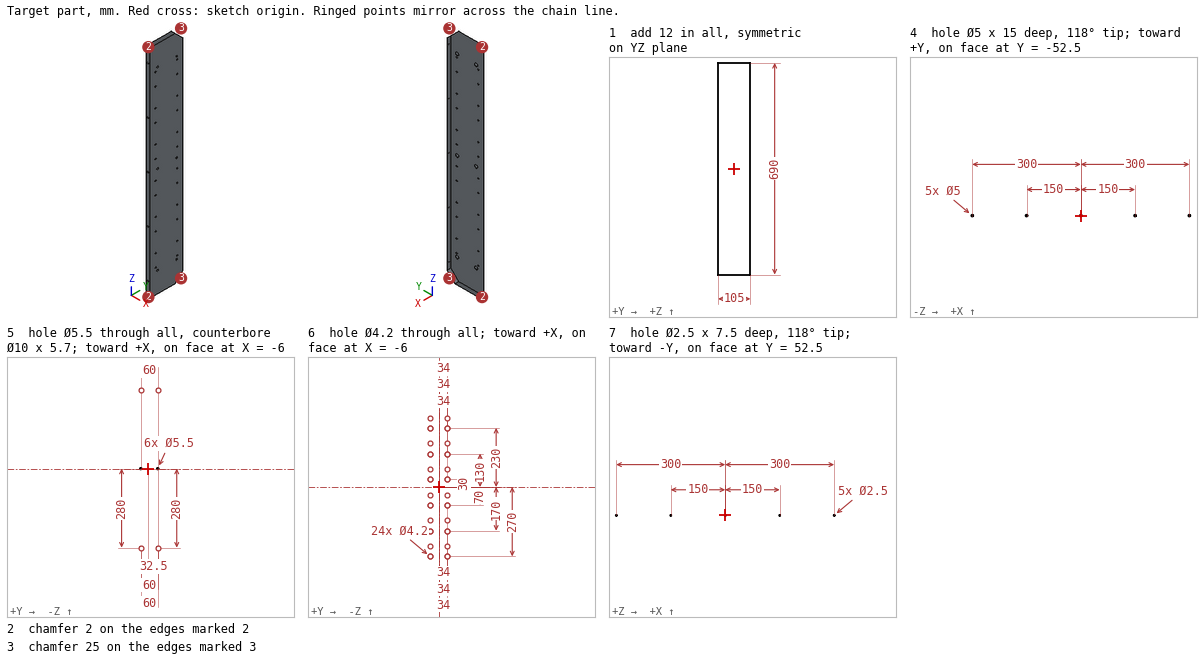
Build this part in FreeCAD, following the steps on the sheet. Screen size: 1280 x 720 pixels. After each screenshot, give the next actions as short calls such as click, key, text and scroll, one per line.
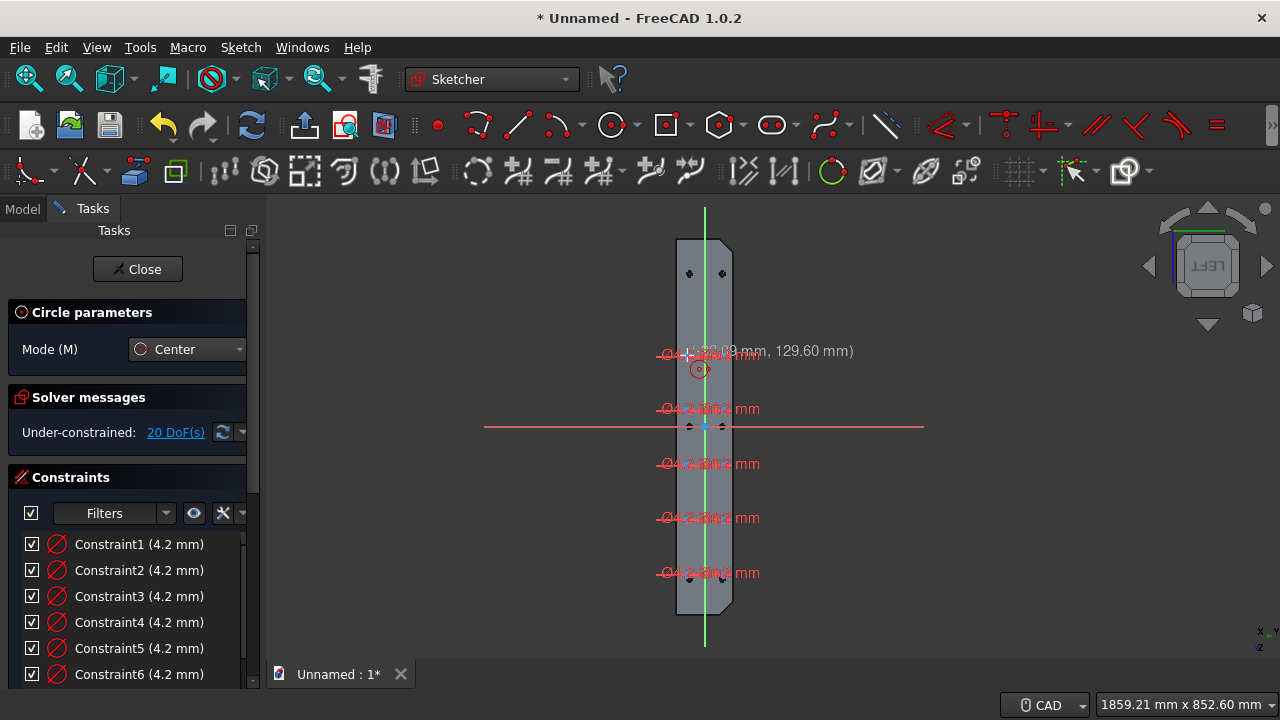
scroll(686, 498, up, 15)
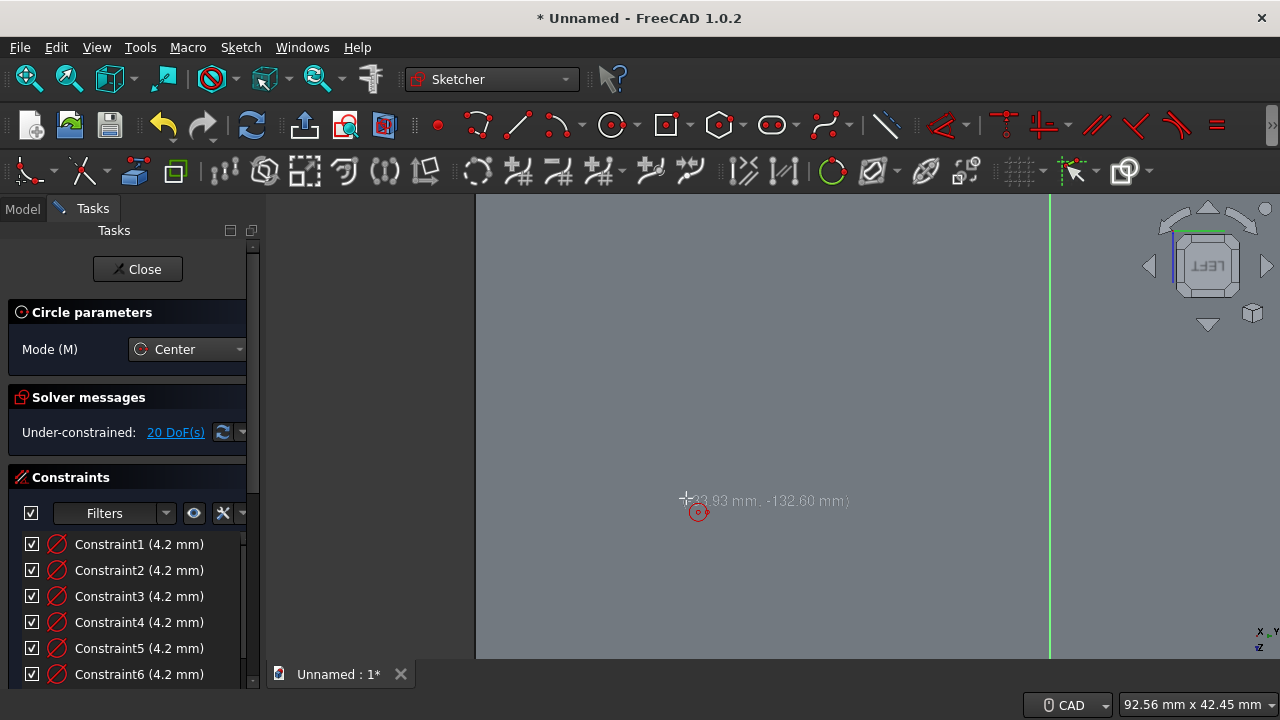
scroll(686, 498, down, 15)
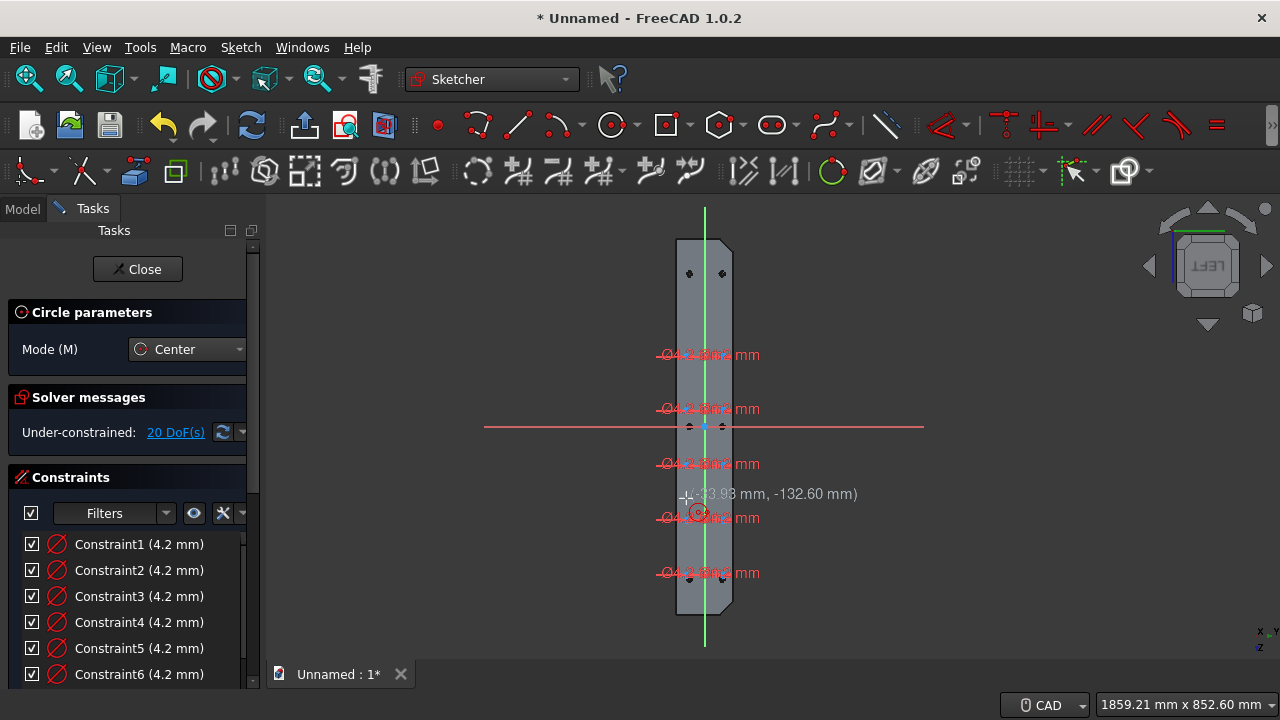
click(686, 498)
move(687, 497)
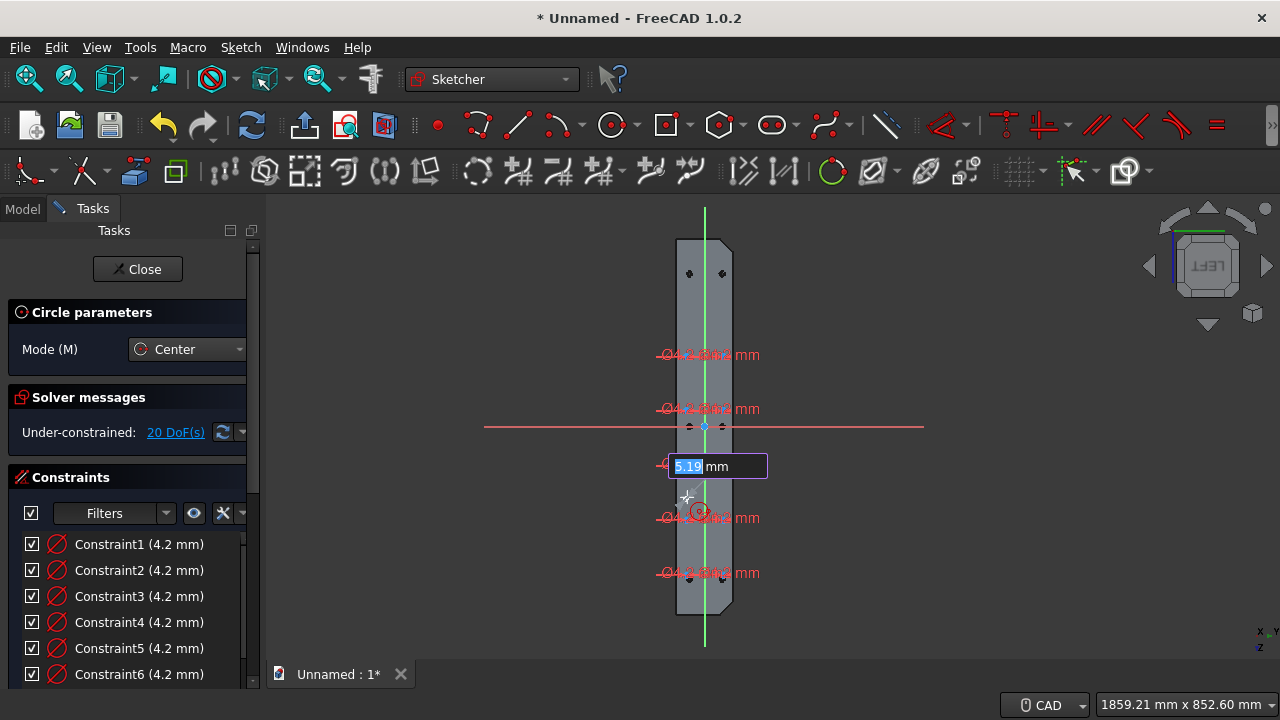
text(4.2)
key(Return)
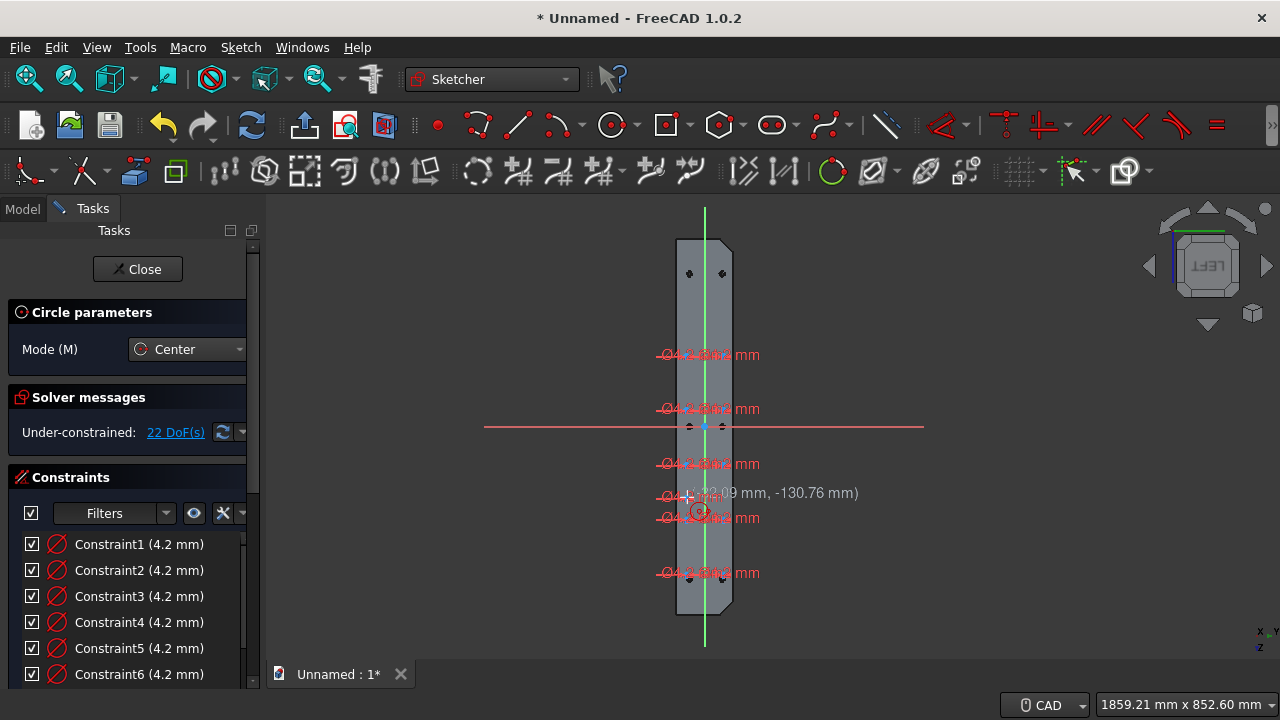
scroll(723, 498, up, 15)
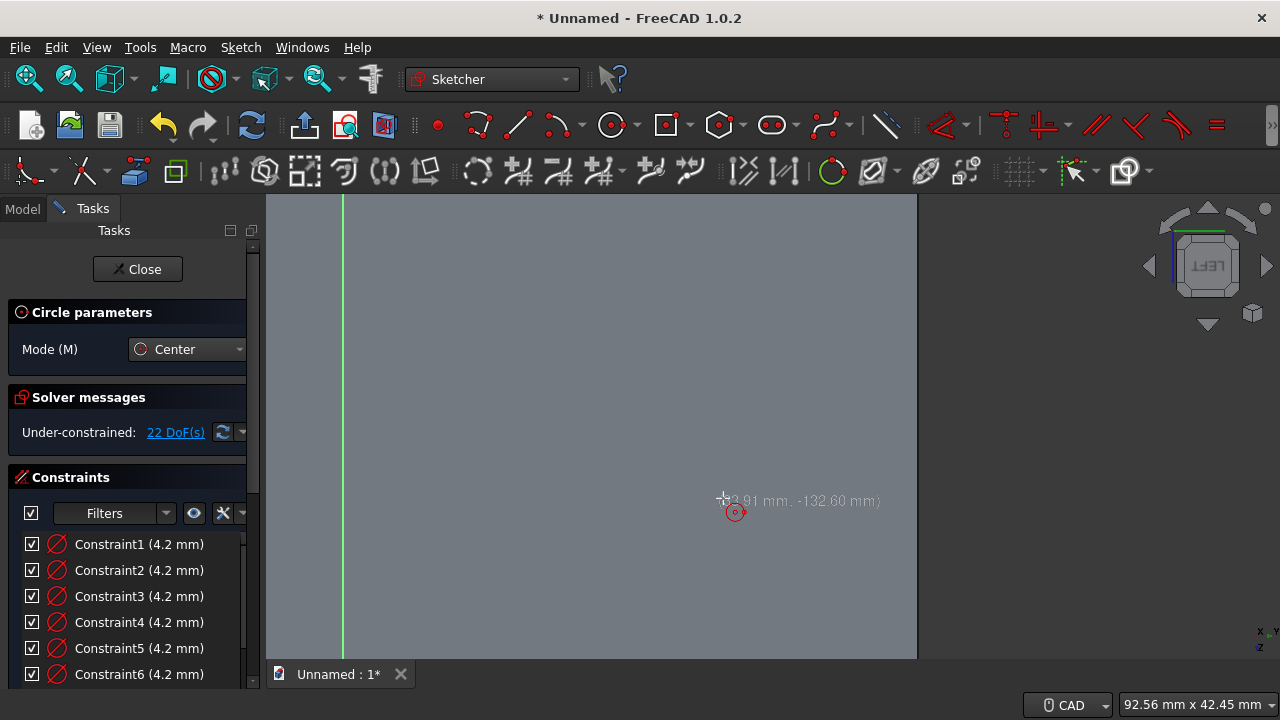
scroll(723, 498, down, 15)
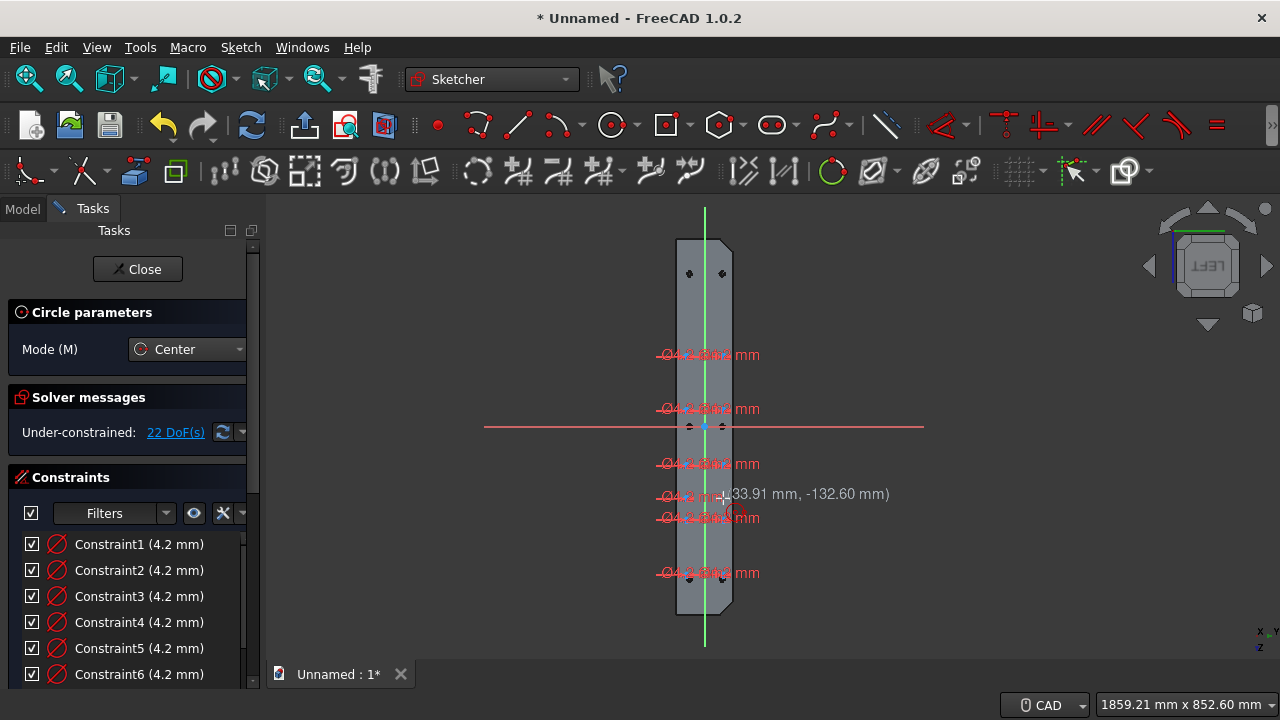
click(723, 498)
move(724, 497)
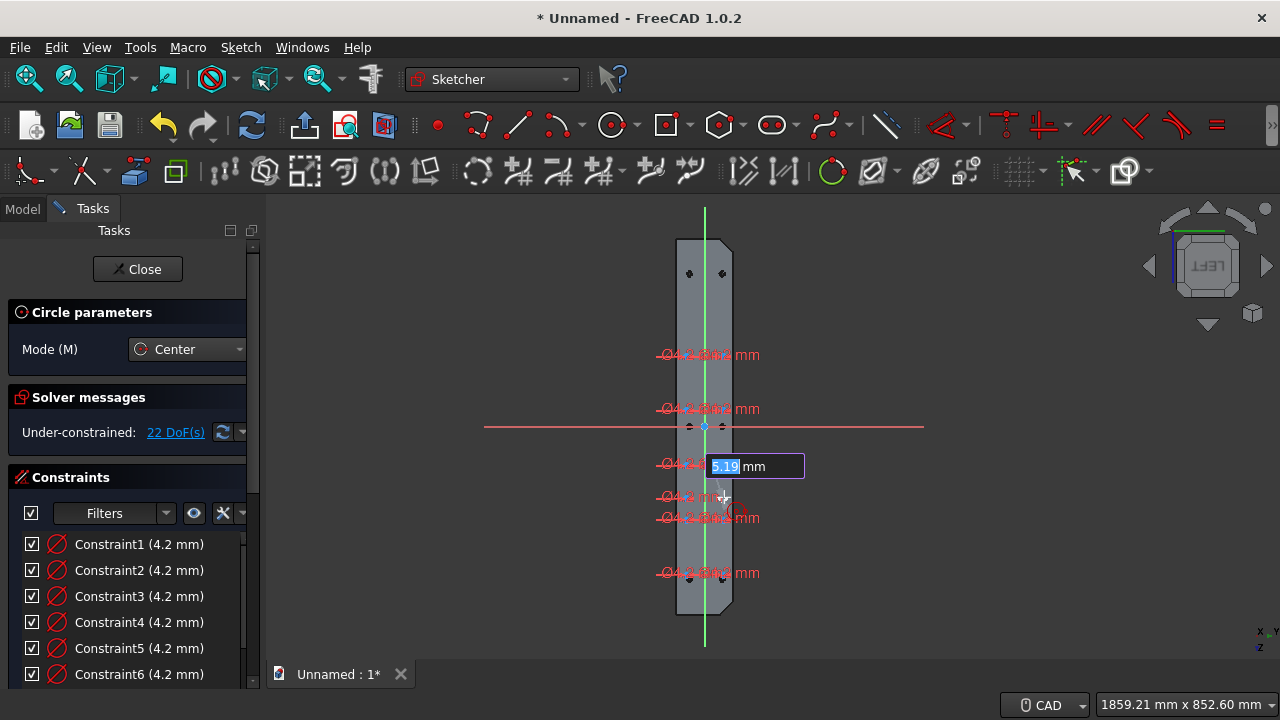
text(4.2)
key(Return)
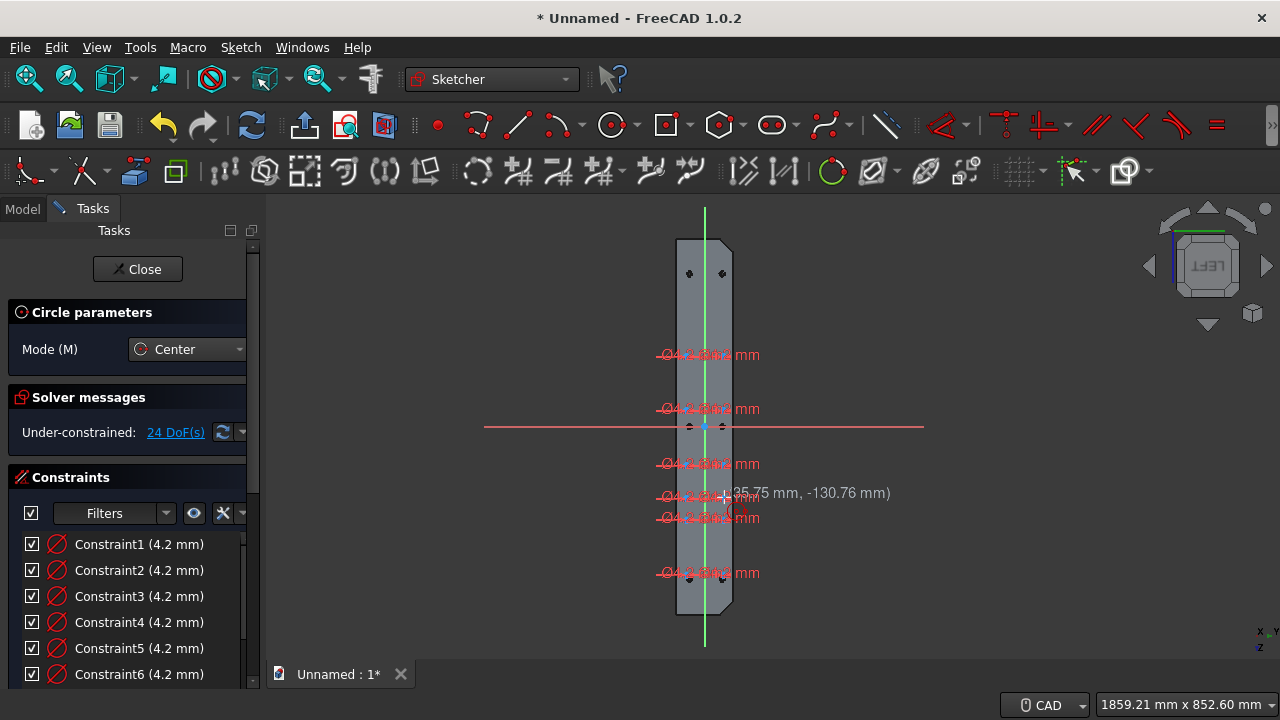
scroll(686, 443, up, 15)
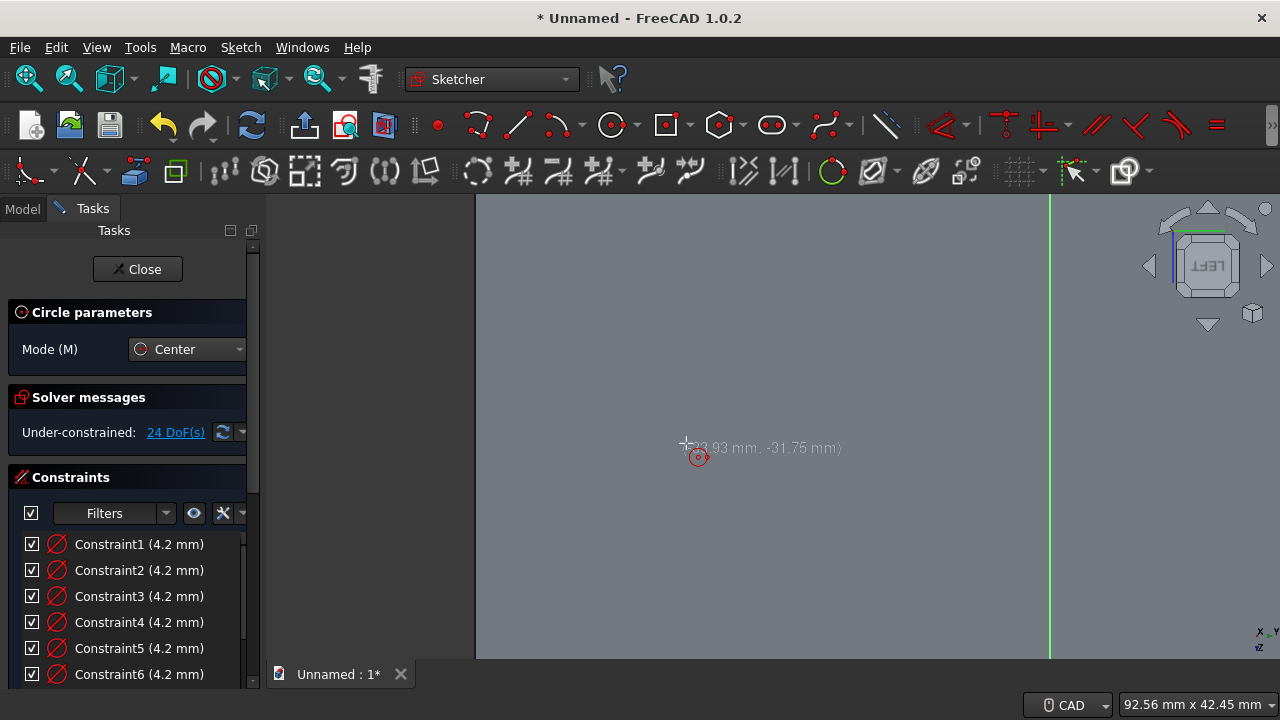
scroll(686, 443, down, 15)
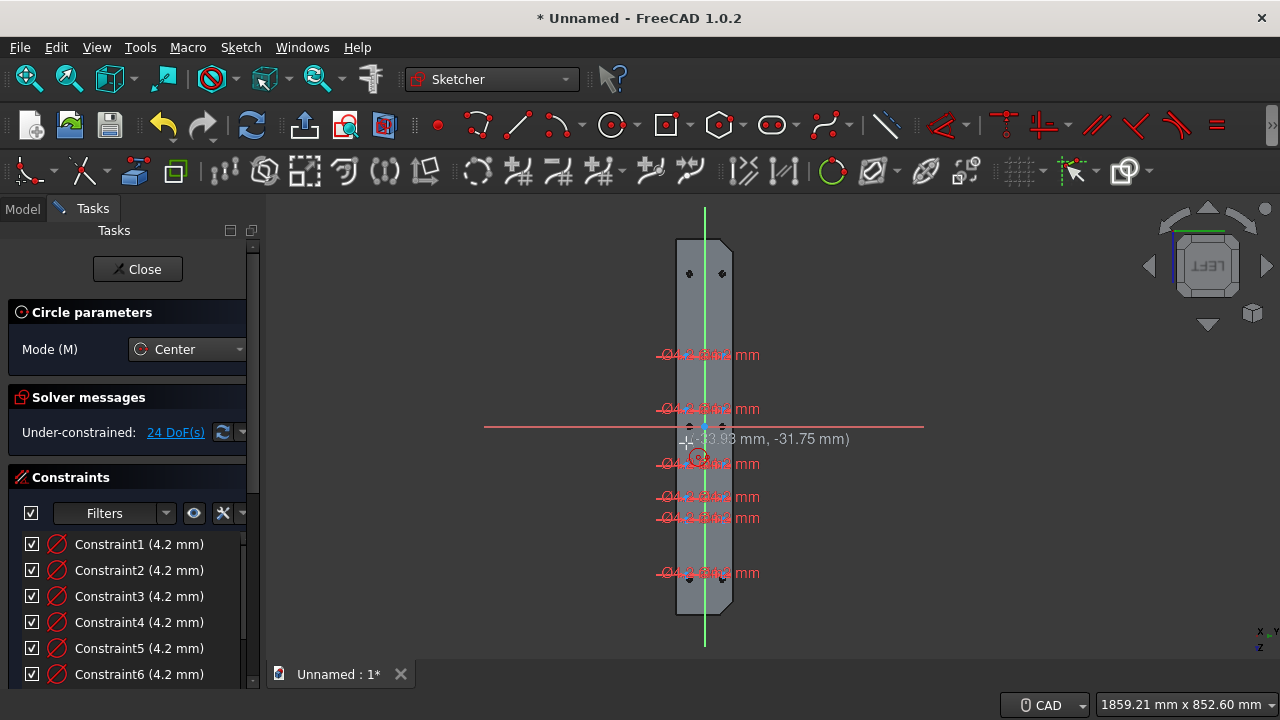
click(686, 443)
move(687, 442)